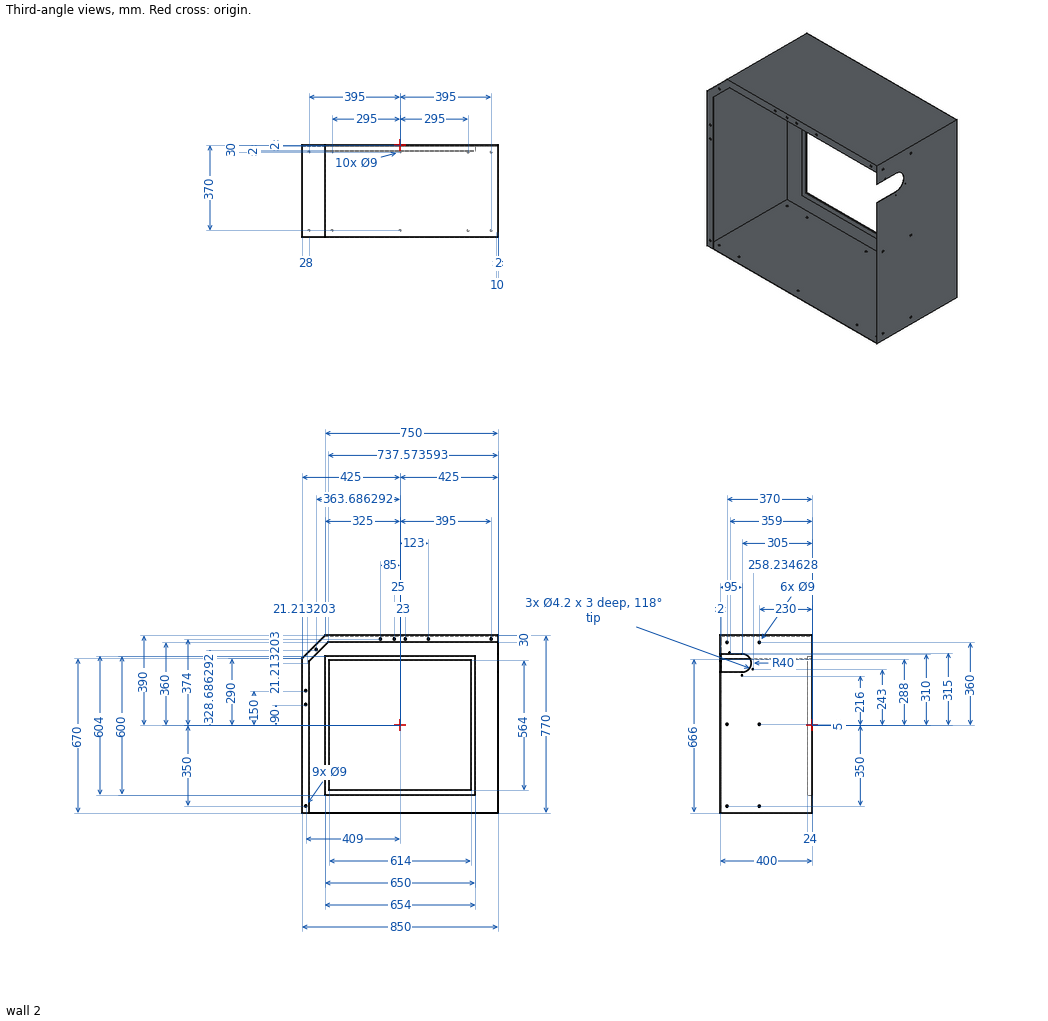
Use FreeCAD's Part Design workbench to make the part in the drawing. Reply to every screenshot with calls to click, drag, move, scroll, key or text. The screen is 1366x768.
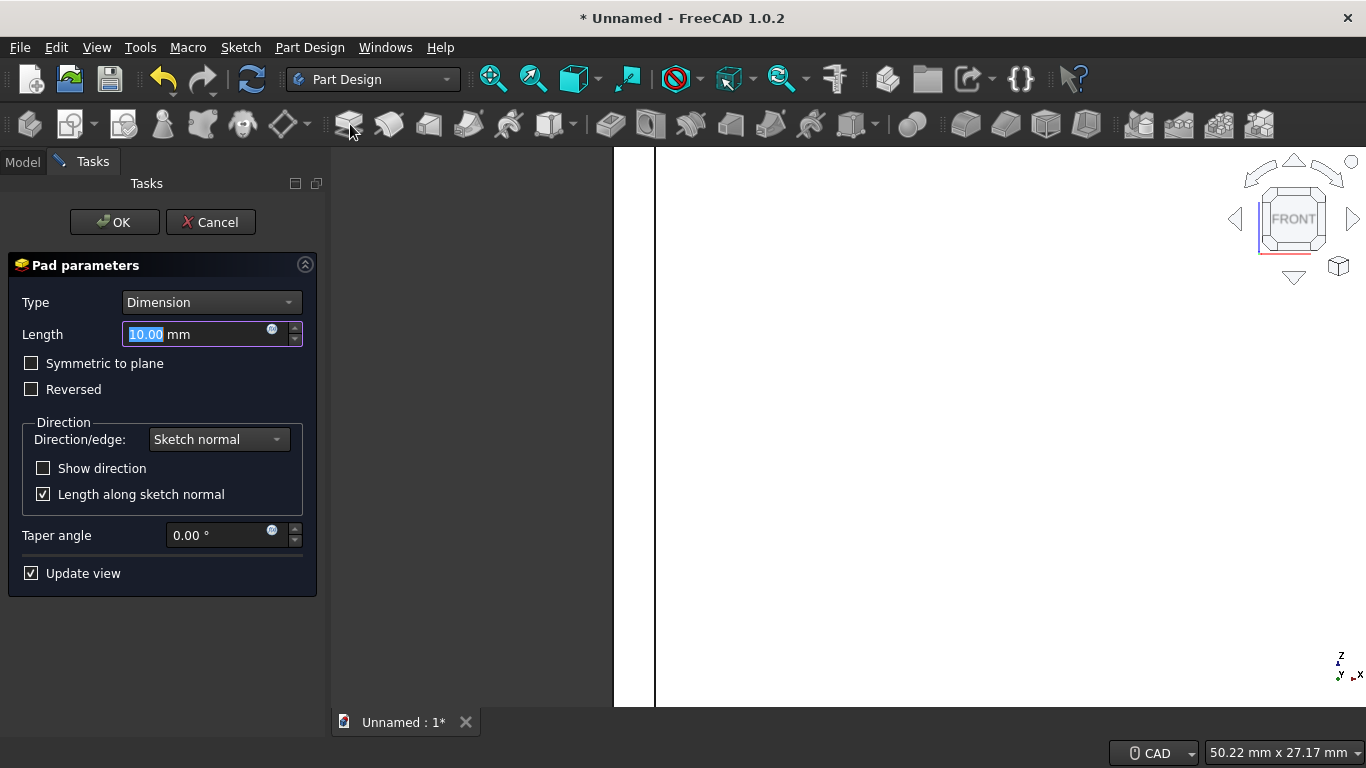
text(2)
key(Tab)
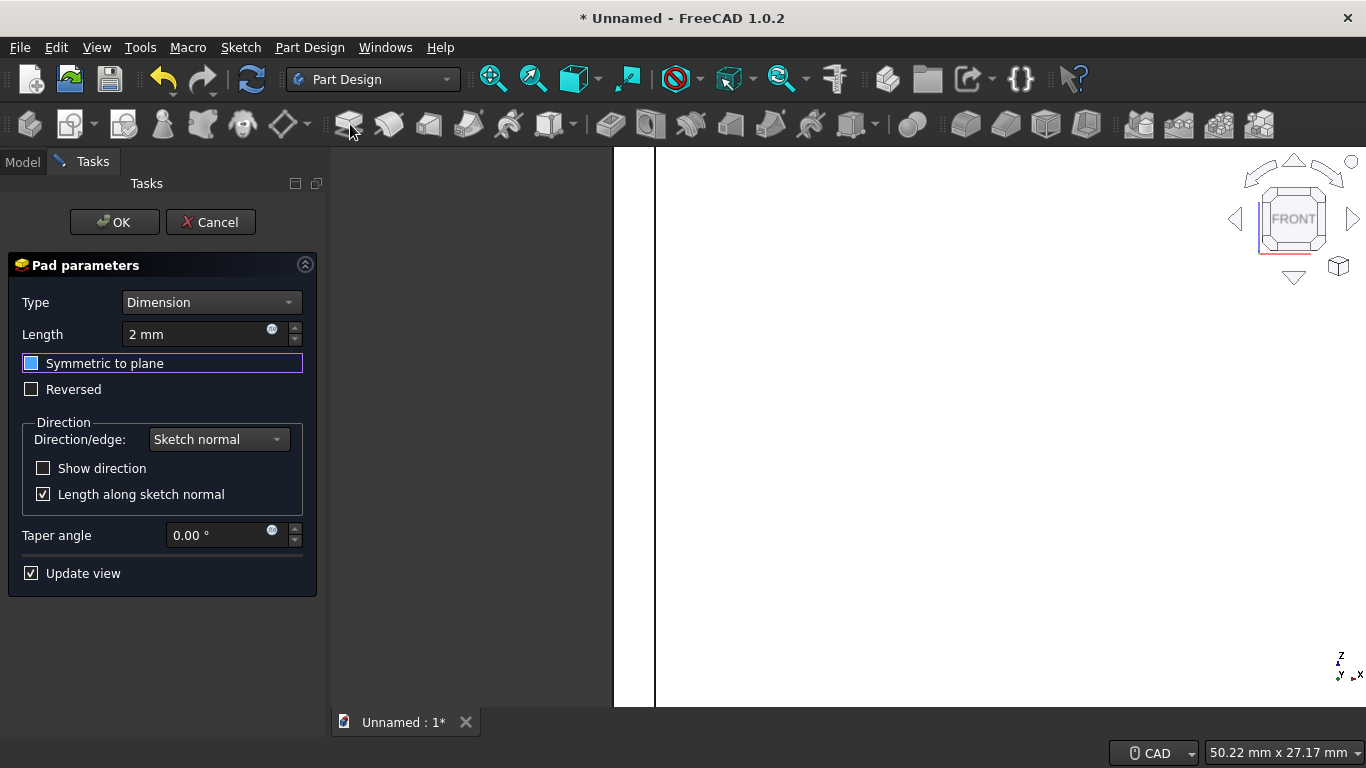
click(30, 389)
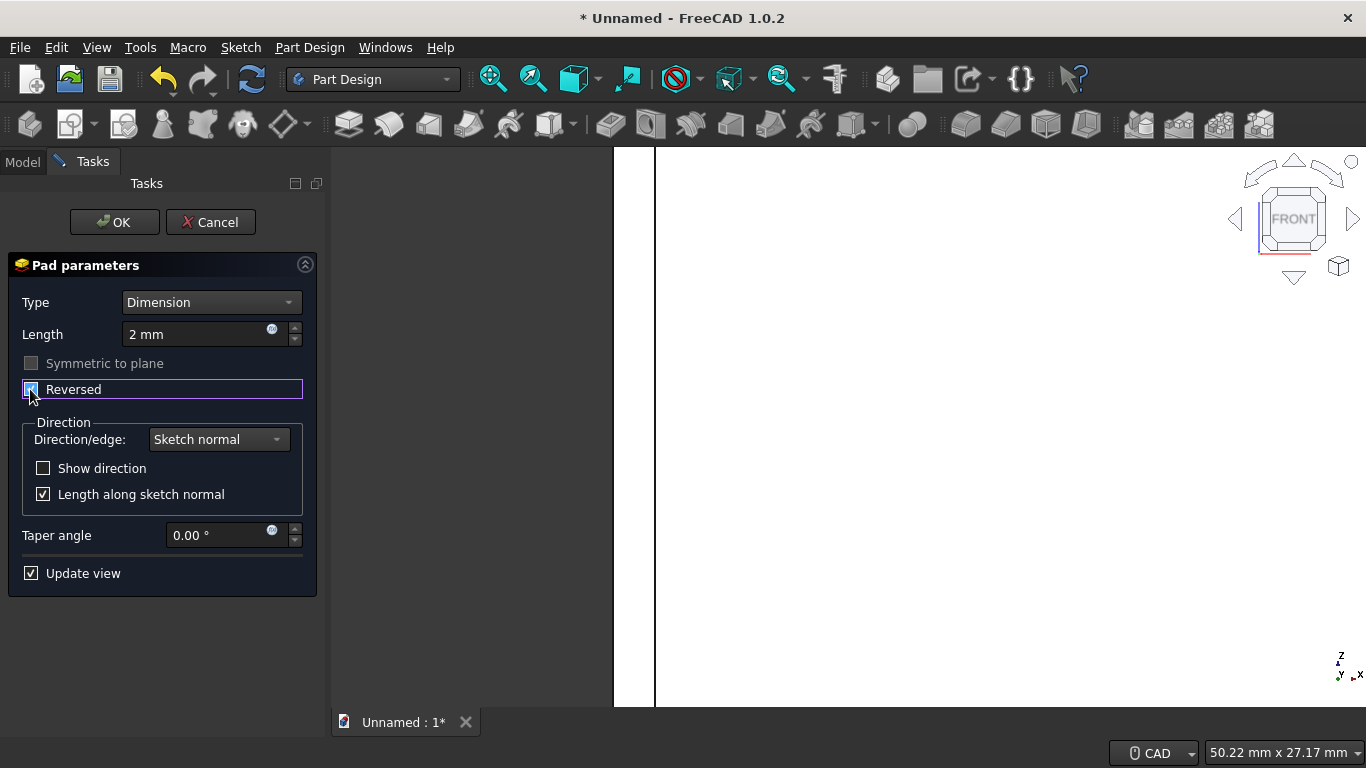
click(115, 222)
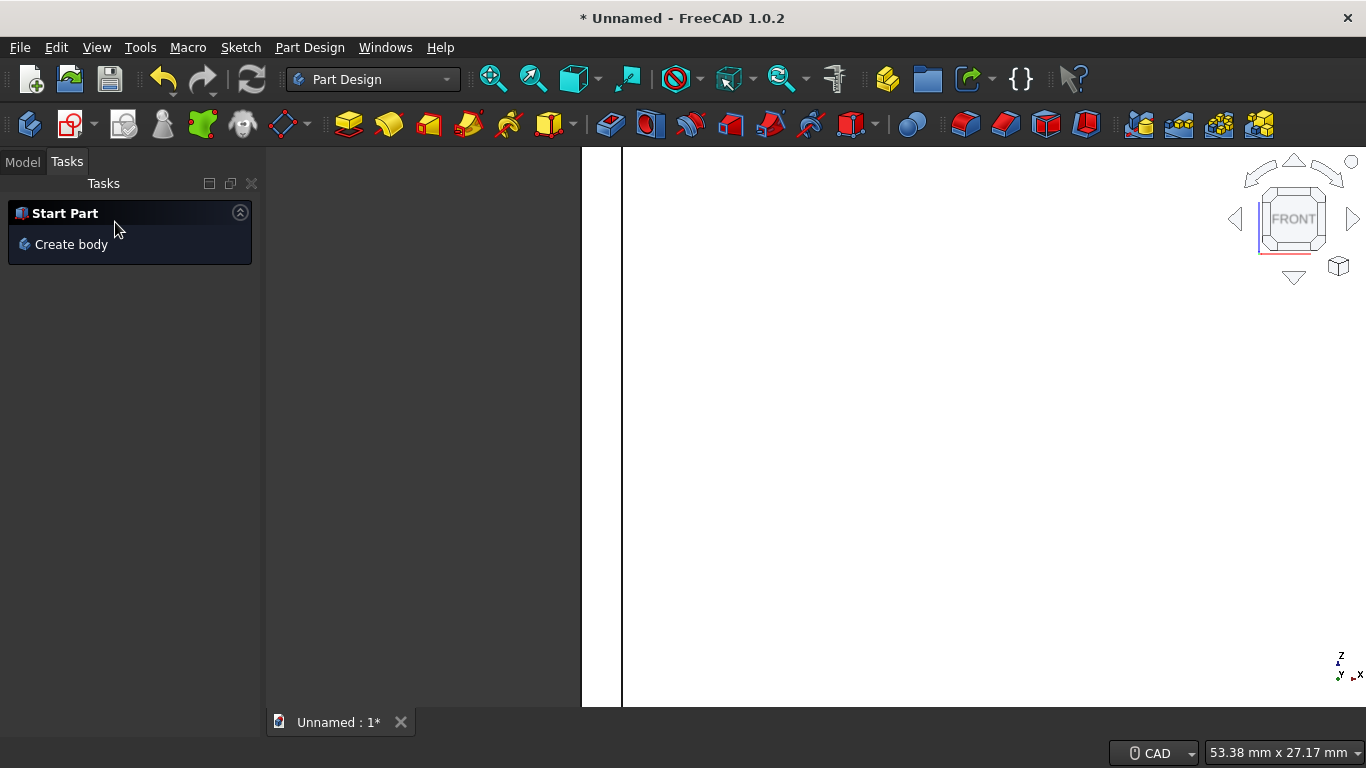
click(494, 80)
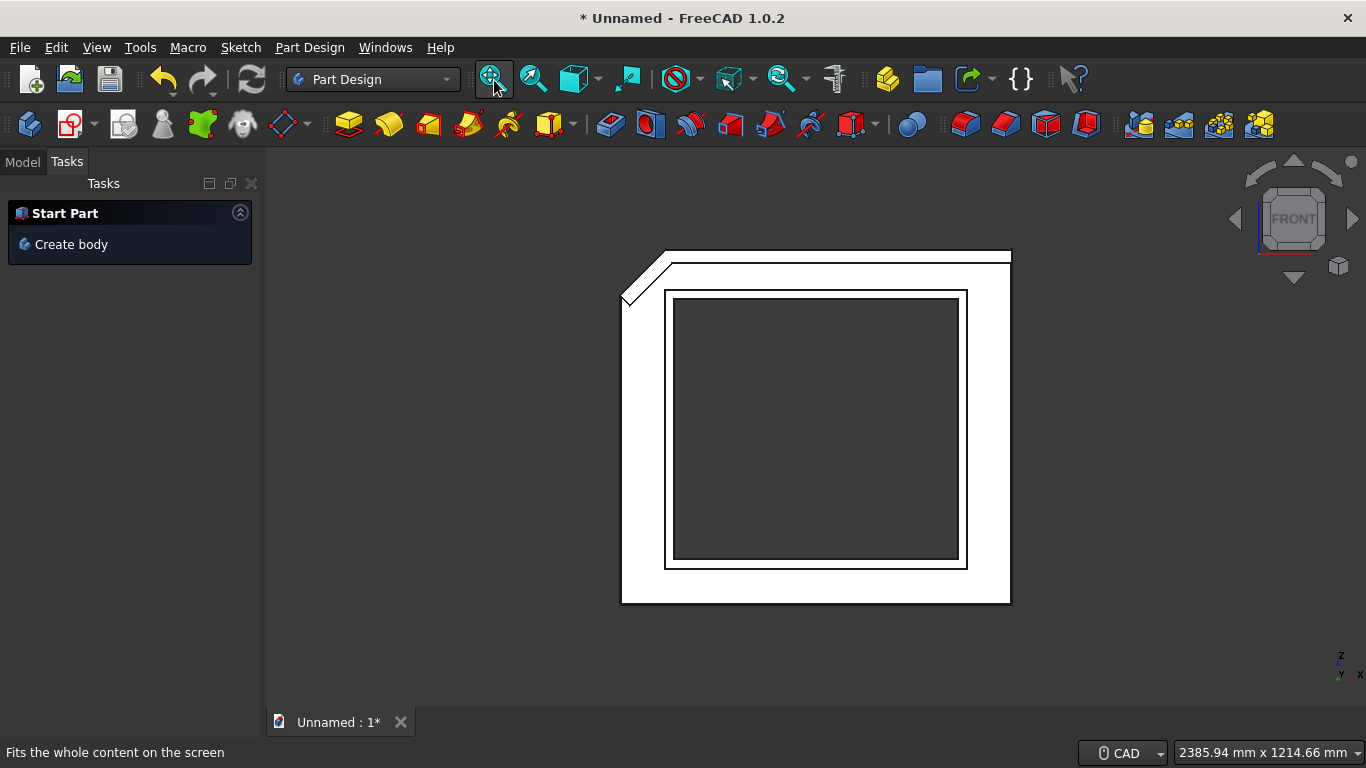
key(0)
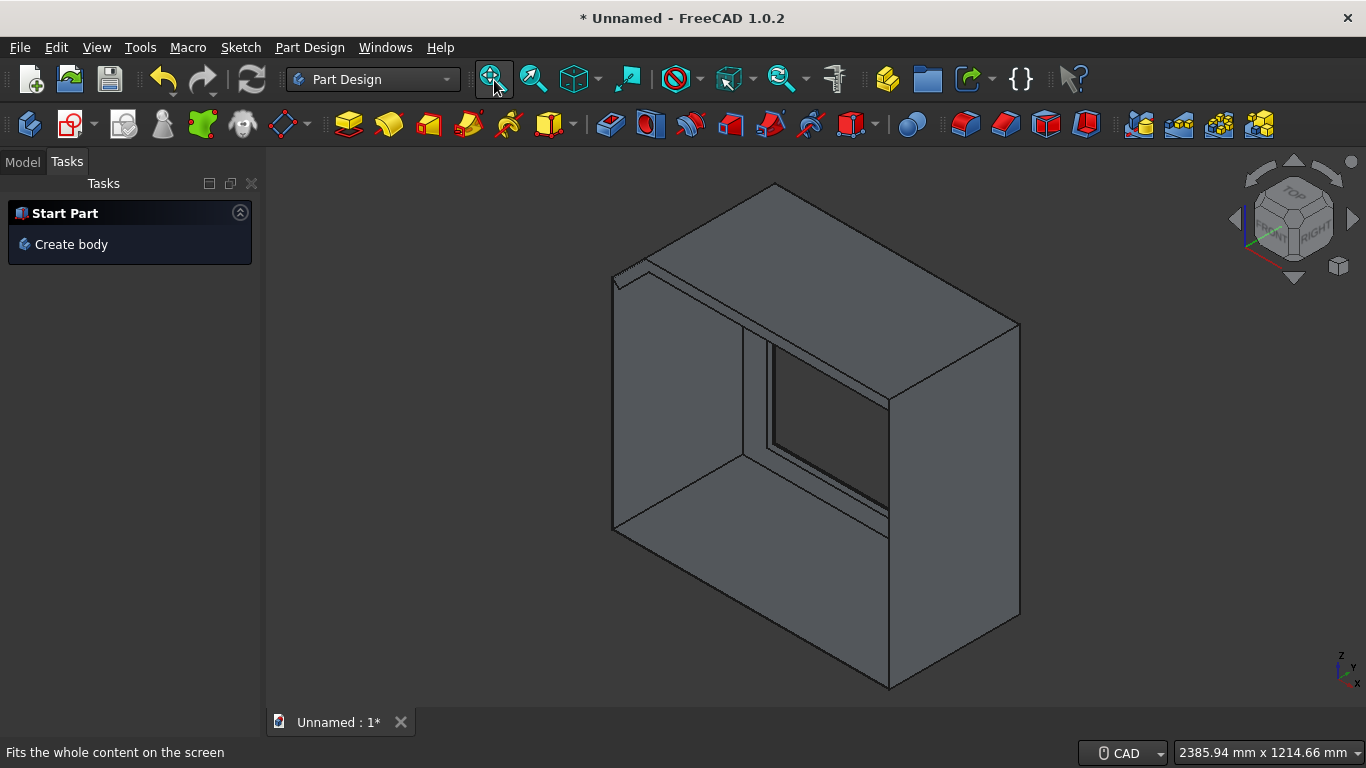
click(955, 506)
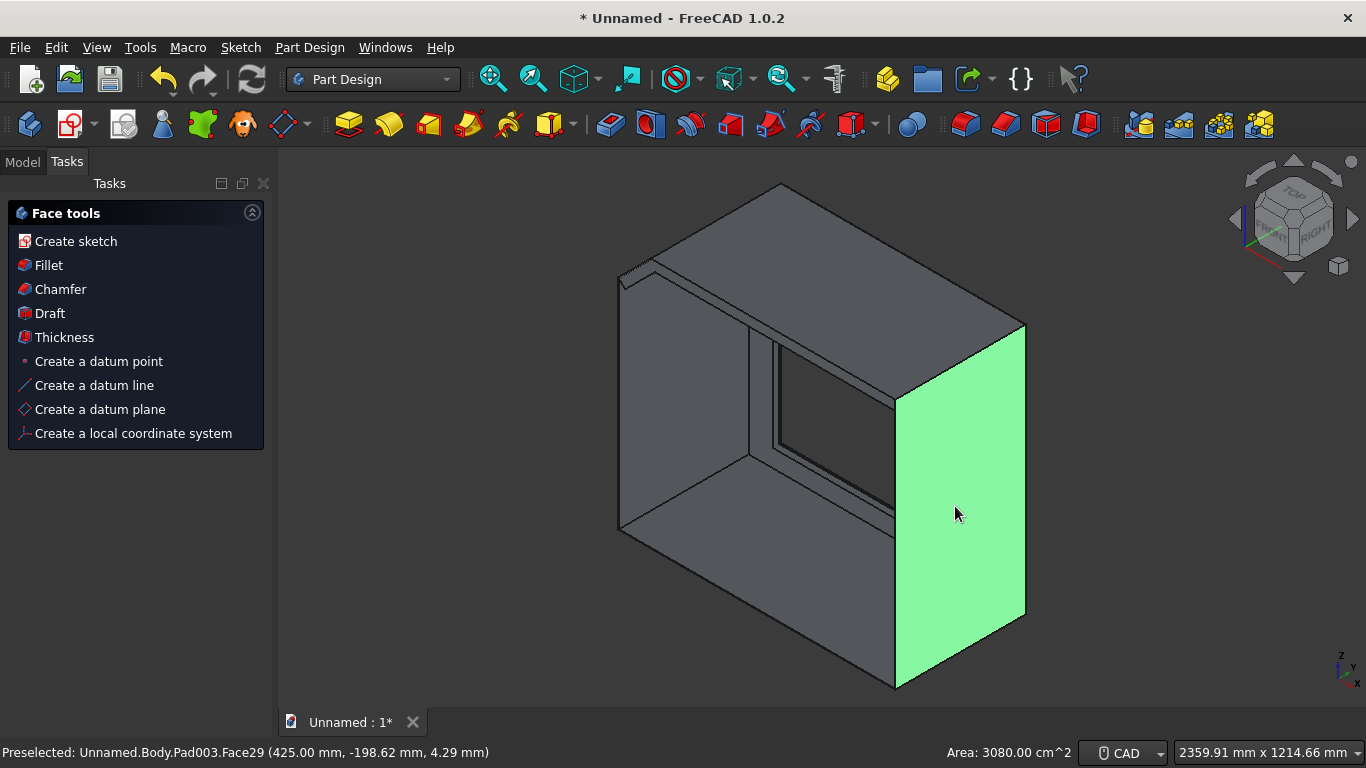
click(70, 124)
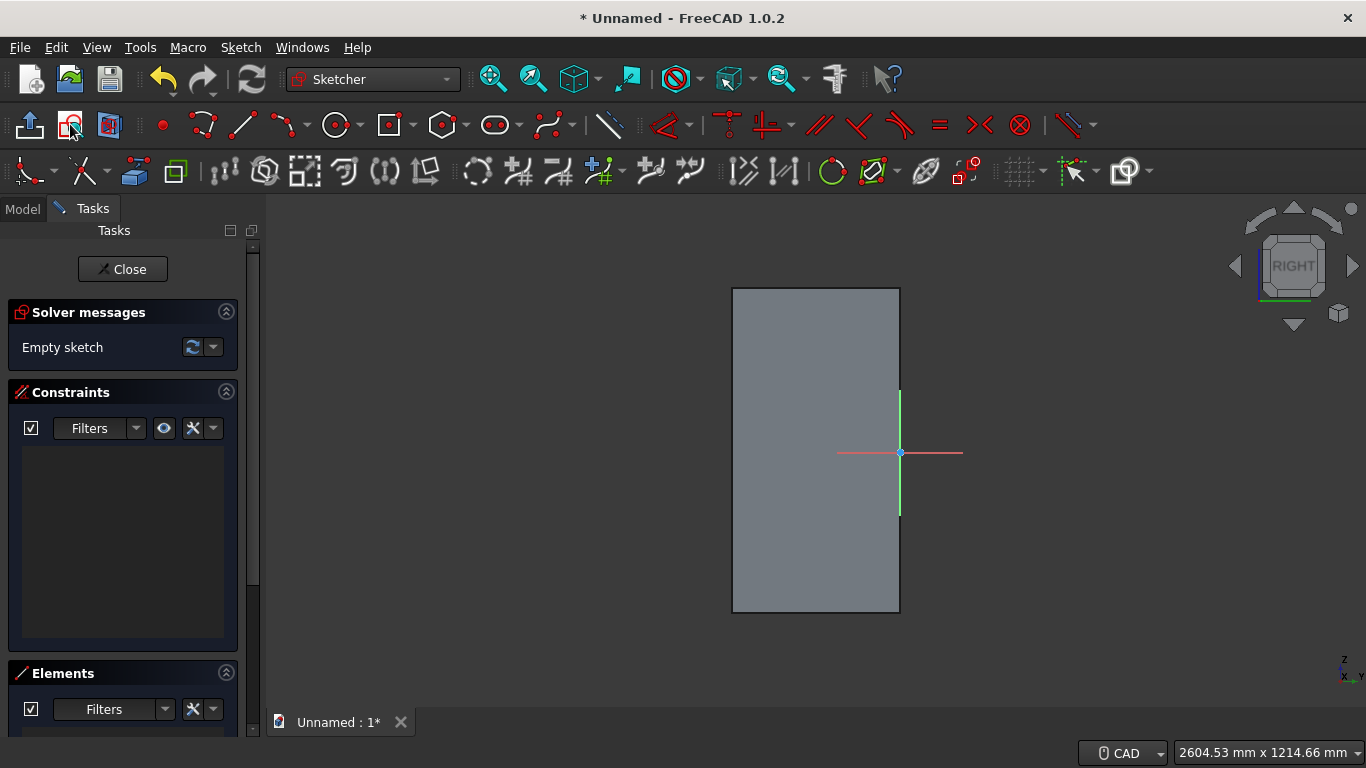
scroll(762, 325, up, 11)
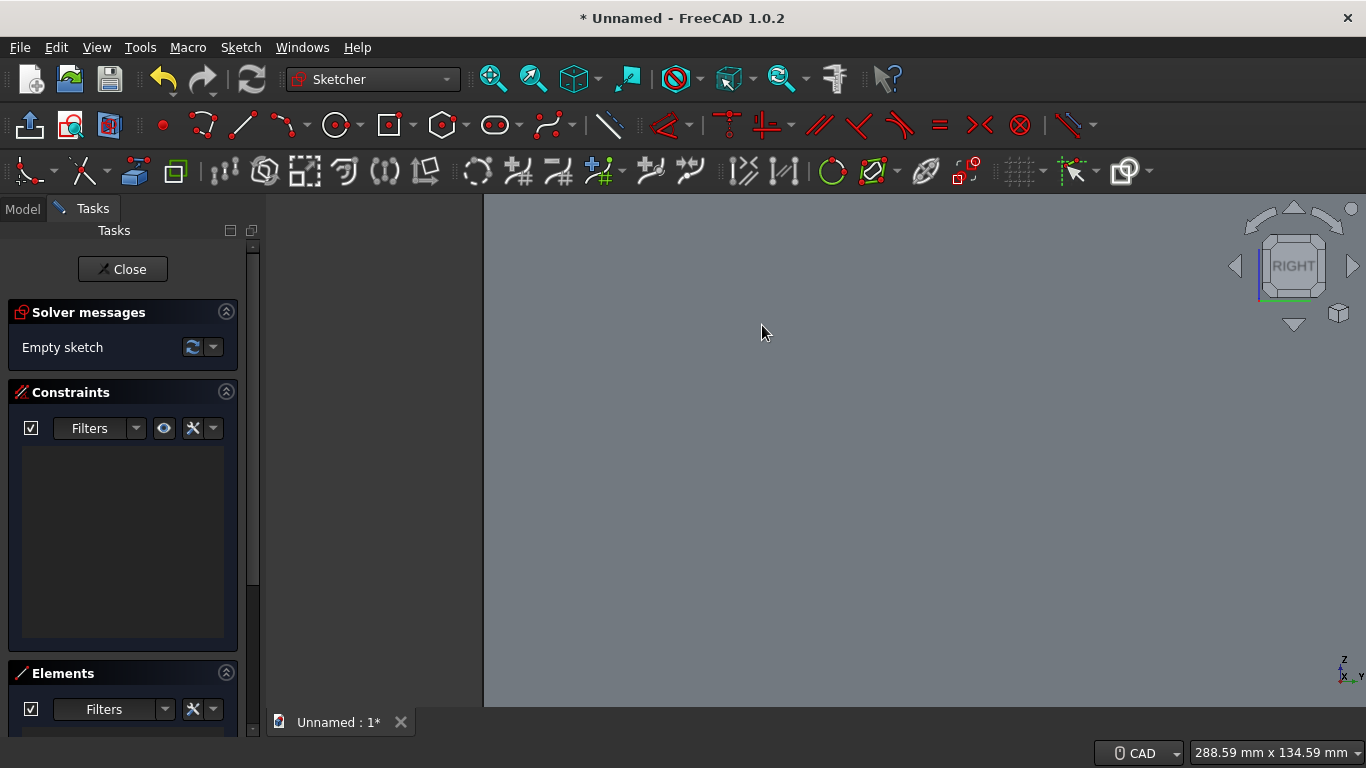
click(204, 126)